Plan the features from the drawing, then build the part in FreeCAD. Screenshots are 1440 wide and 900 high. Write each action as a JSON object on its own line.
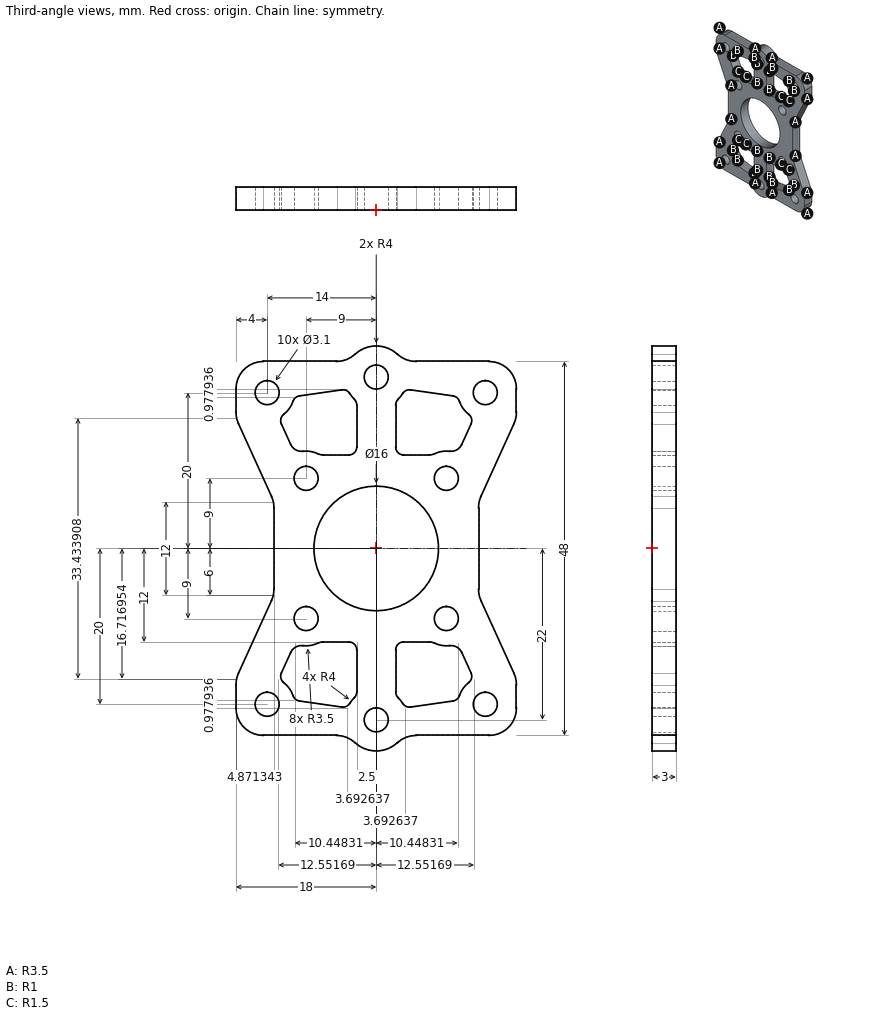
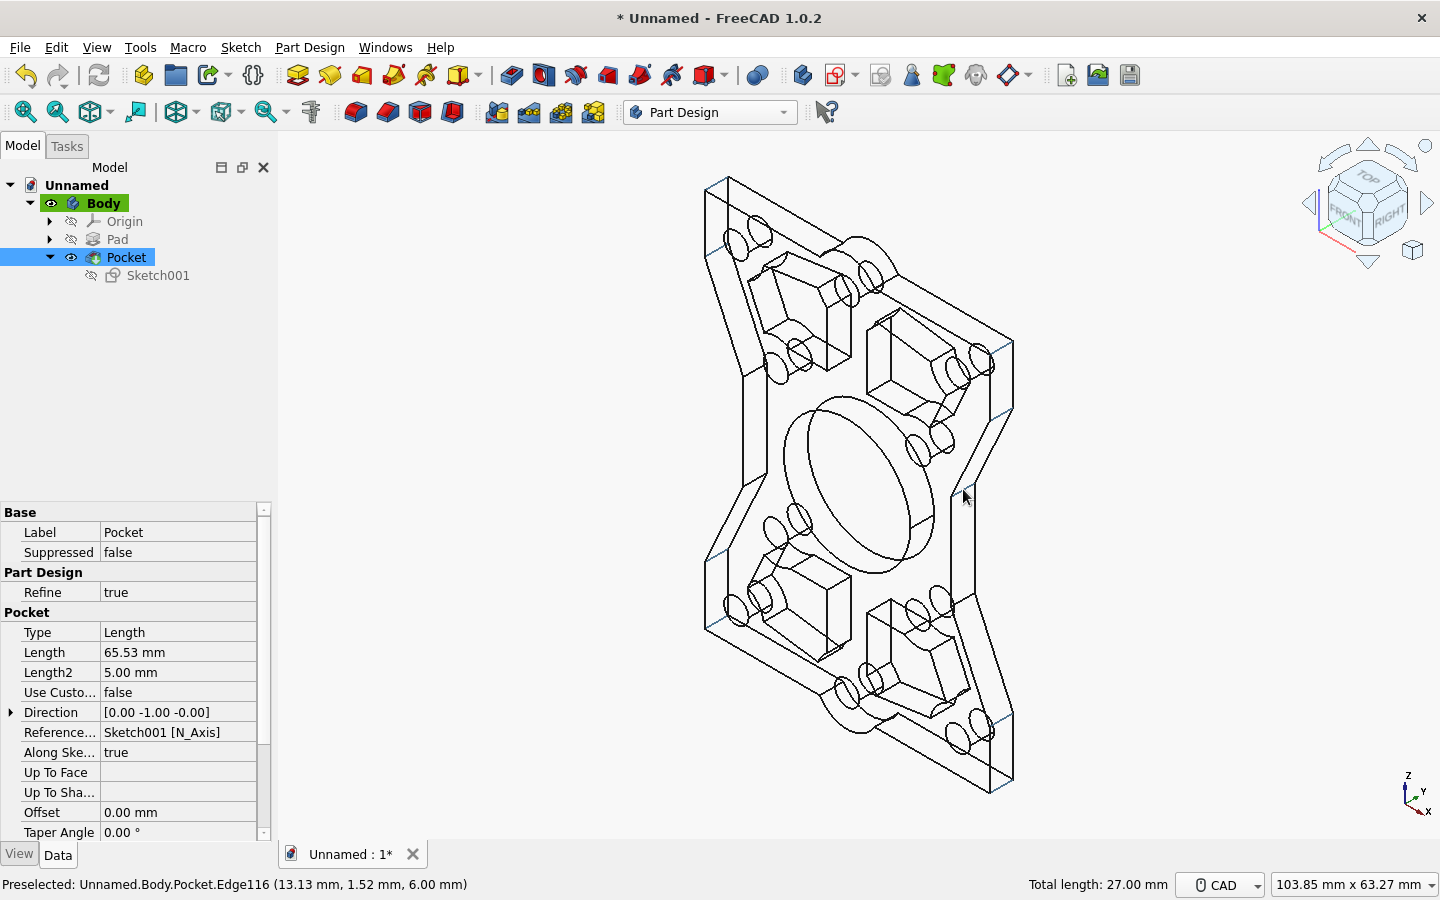
{"action": "left_click", "coordinate": [963, 599], "text": "ctrl"}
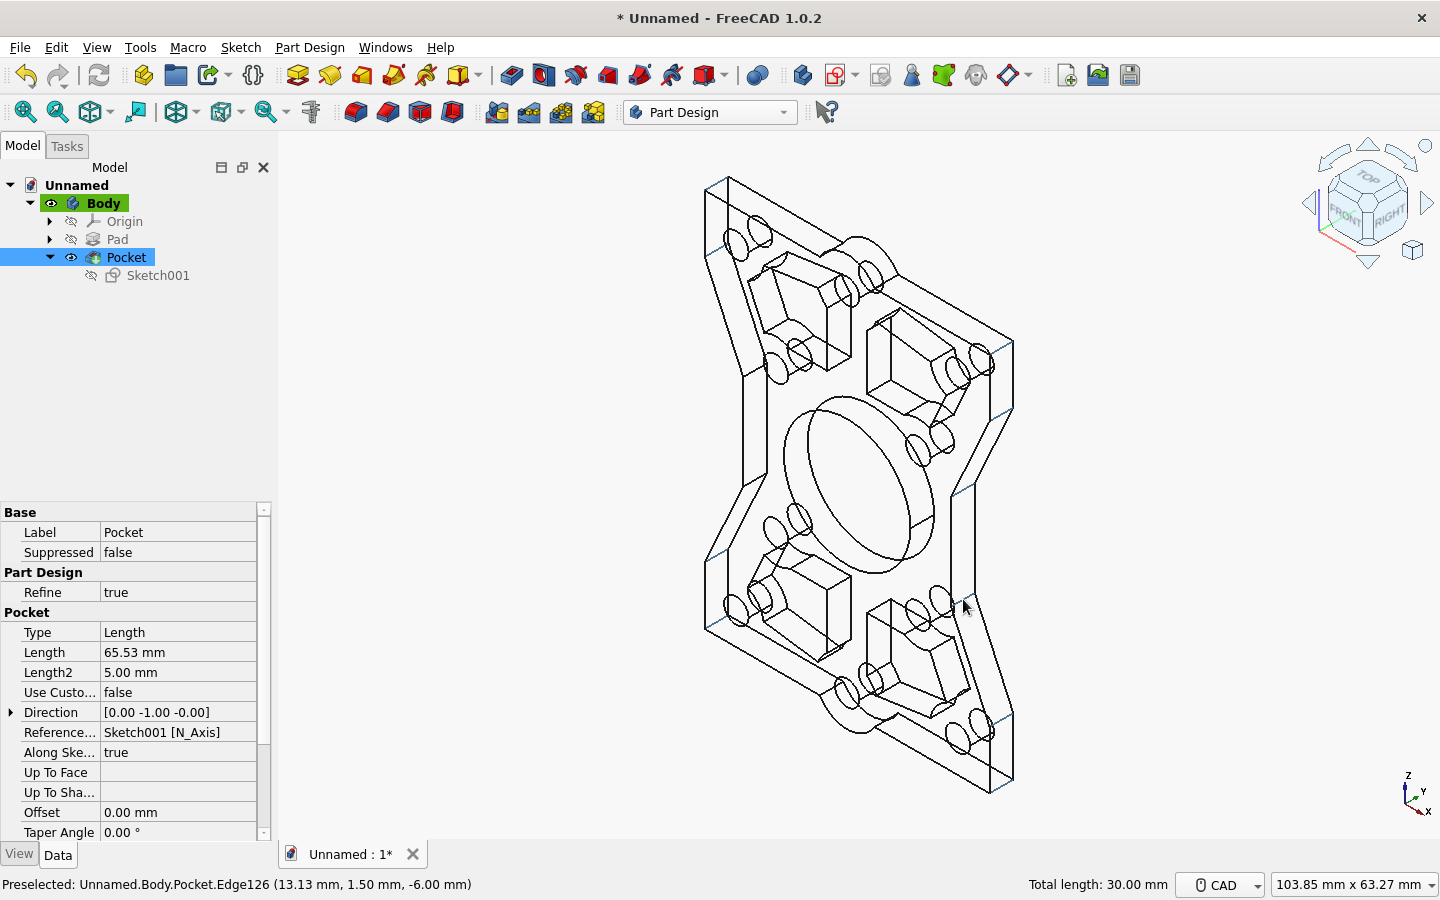
{"action": "left_click", "coordinate": [755, 479], "text": "ctrl"}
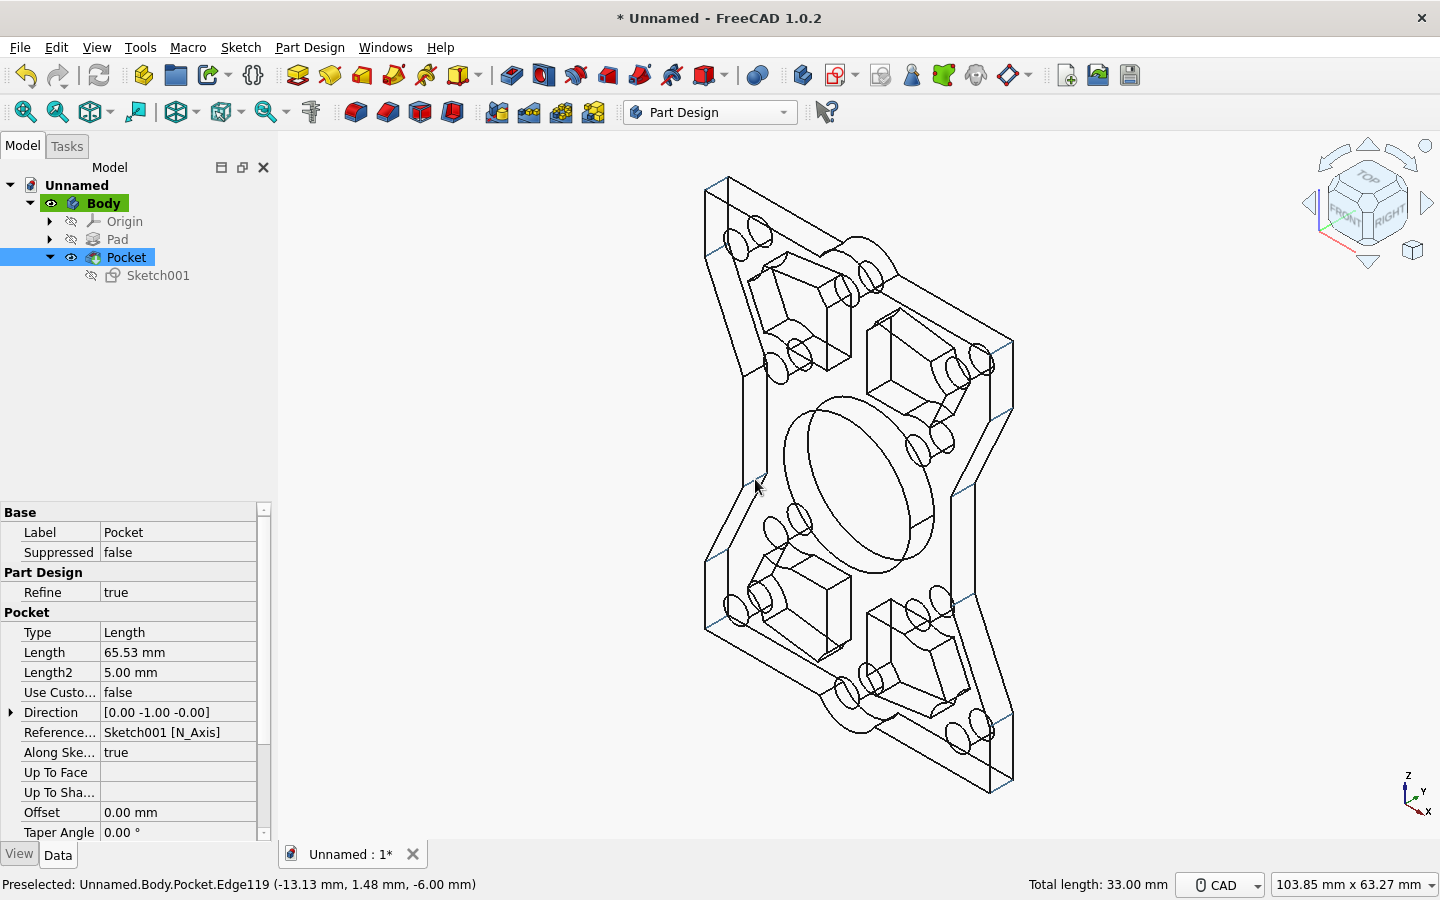
{"action": "left_click", "coordinate": [755, 369], "text": "ctrl"}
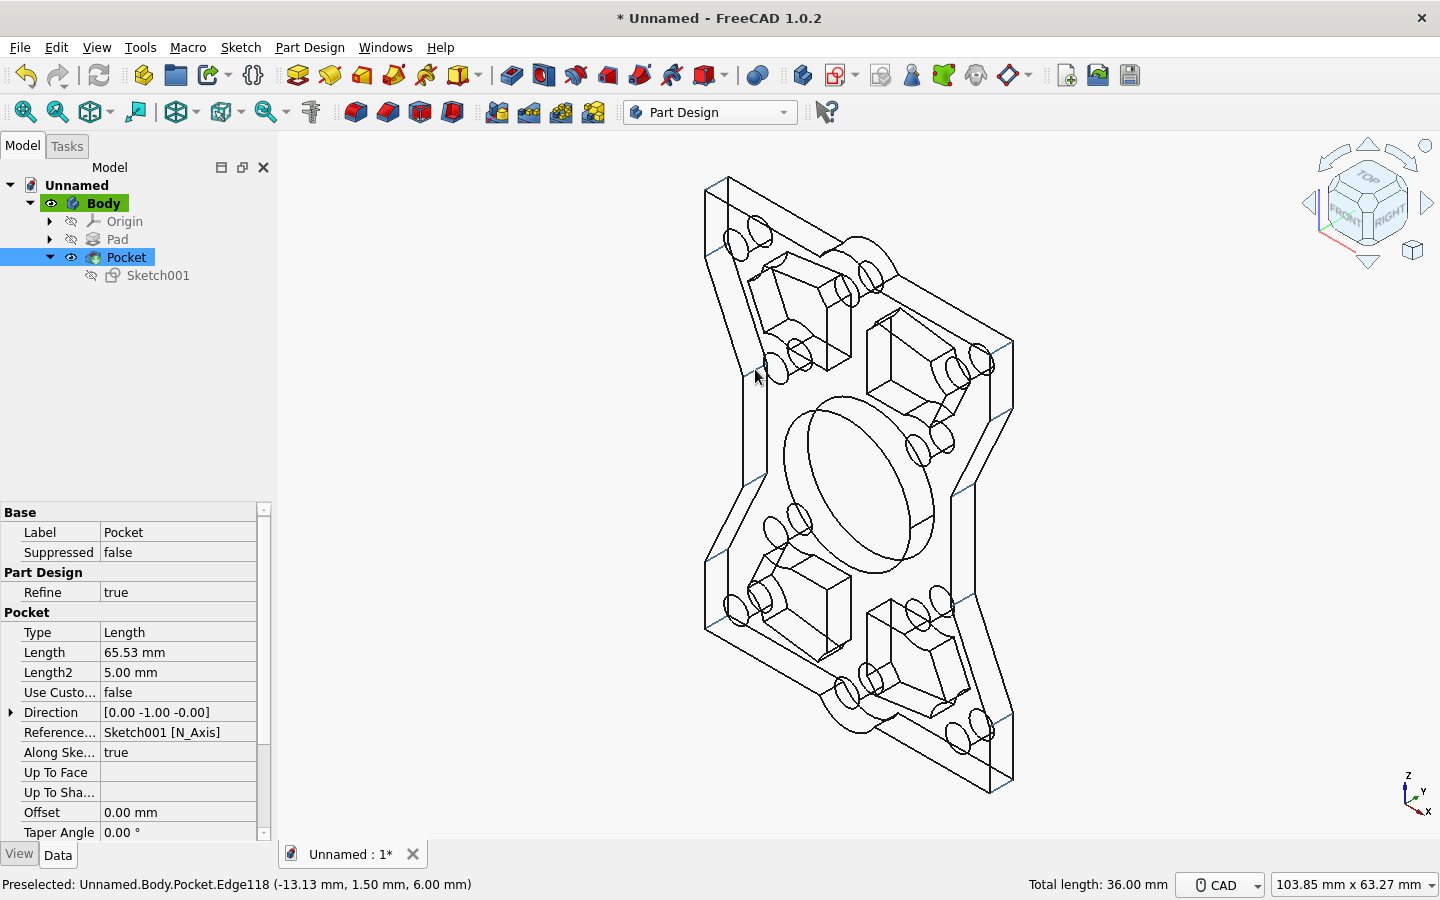
{"action": "left_click", "coordinate": [829, 689], "text": "ctrl"}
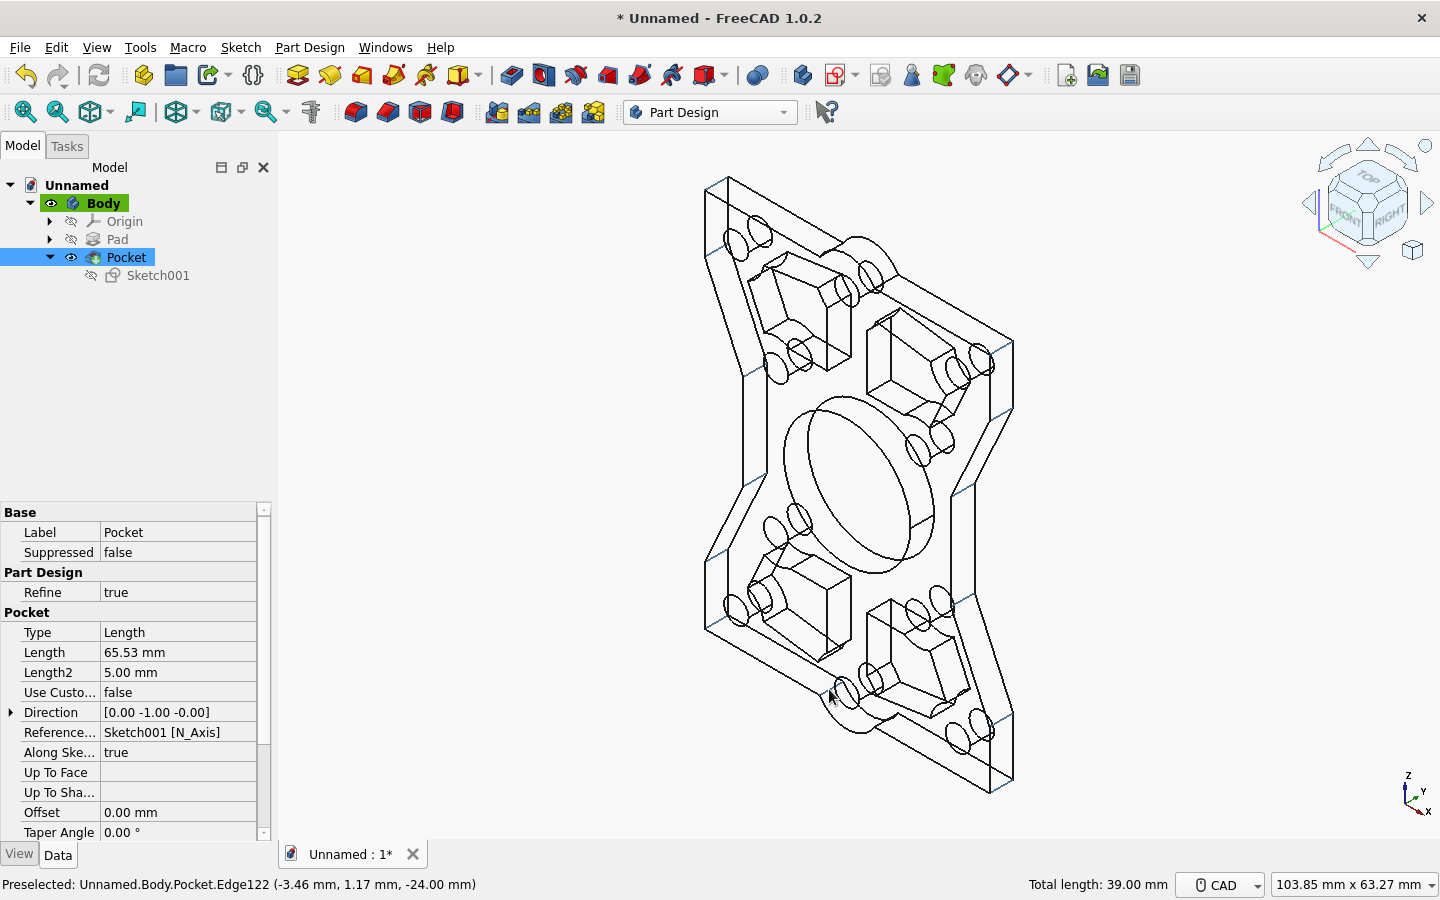
{"action": "left_click", "coordinate": [886, 719], "text": "ctrl"}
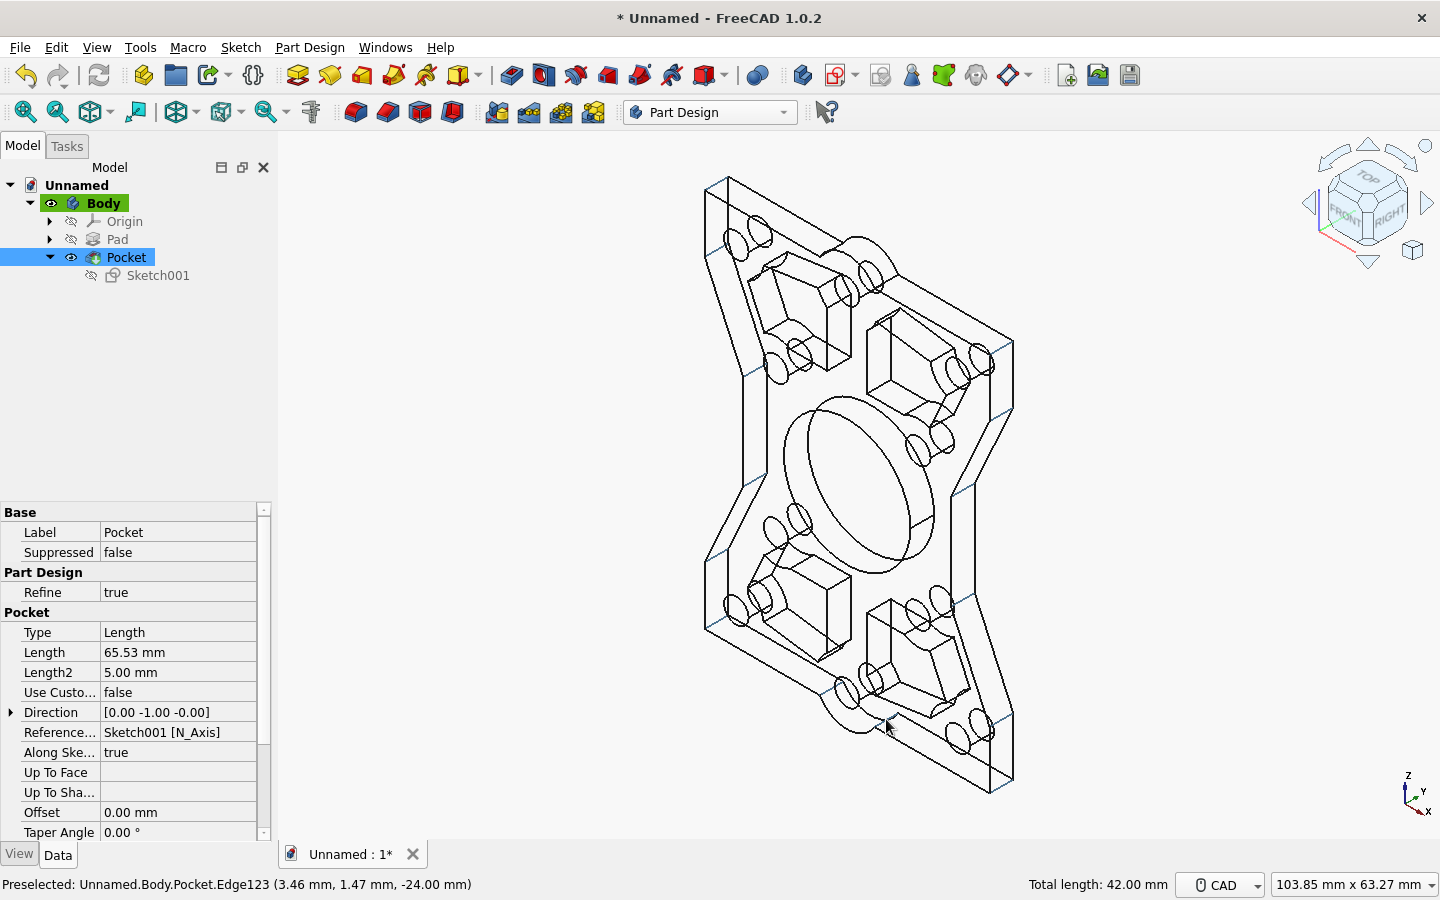
{"action": "left_click", "coordinate": [886, 281], "text": "ctrl"}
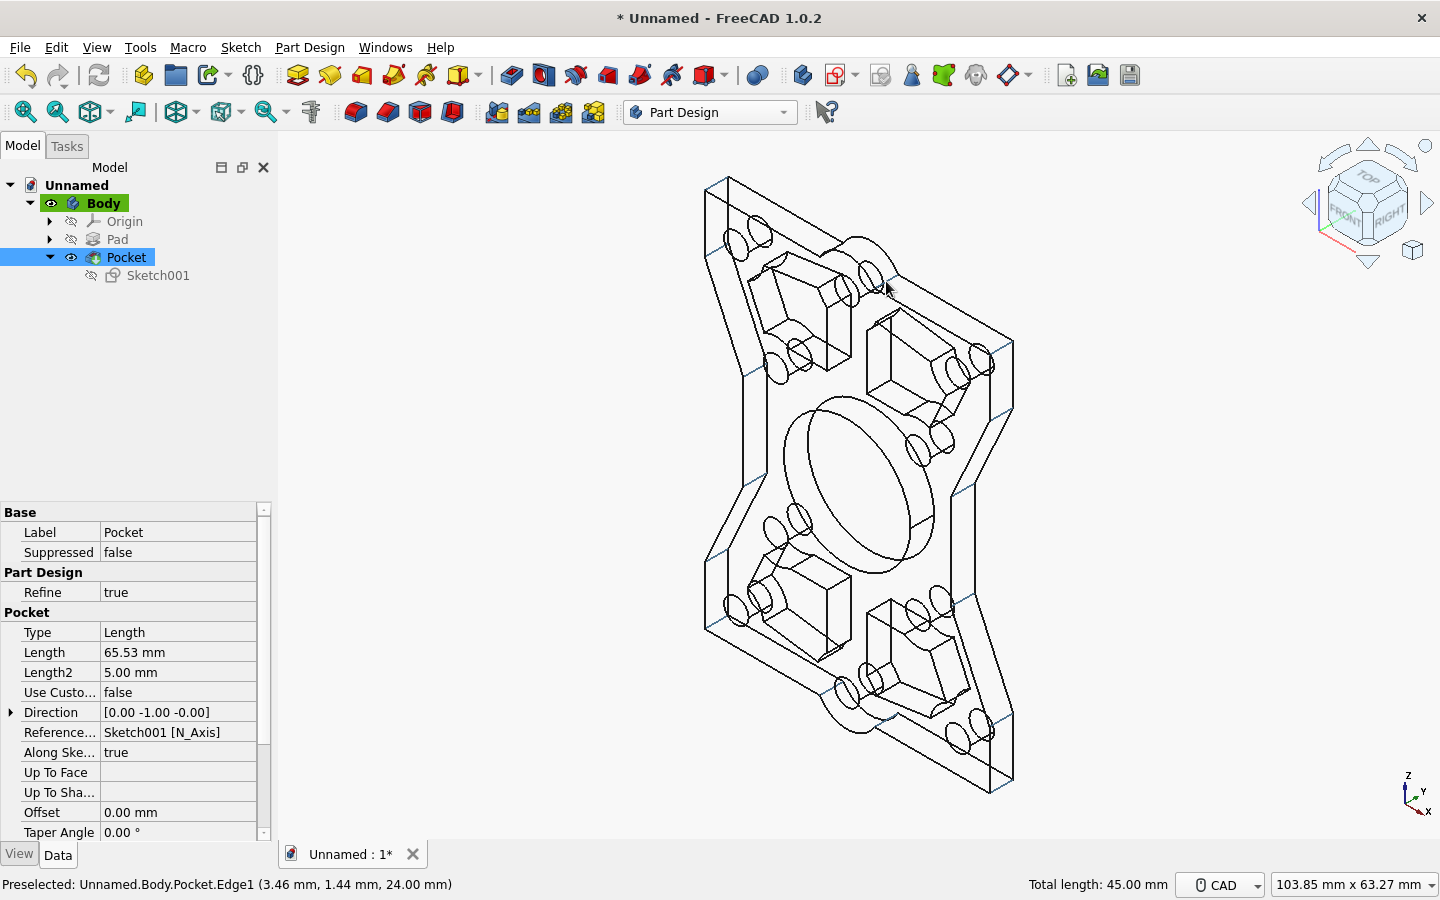
{"action": "key", "text": "2"}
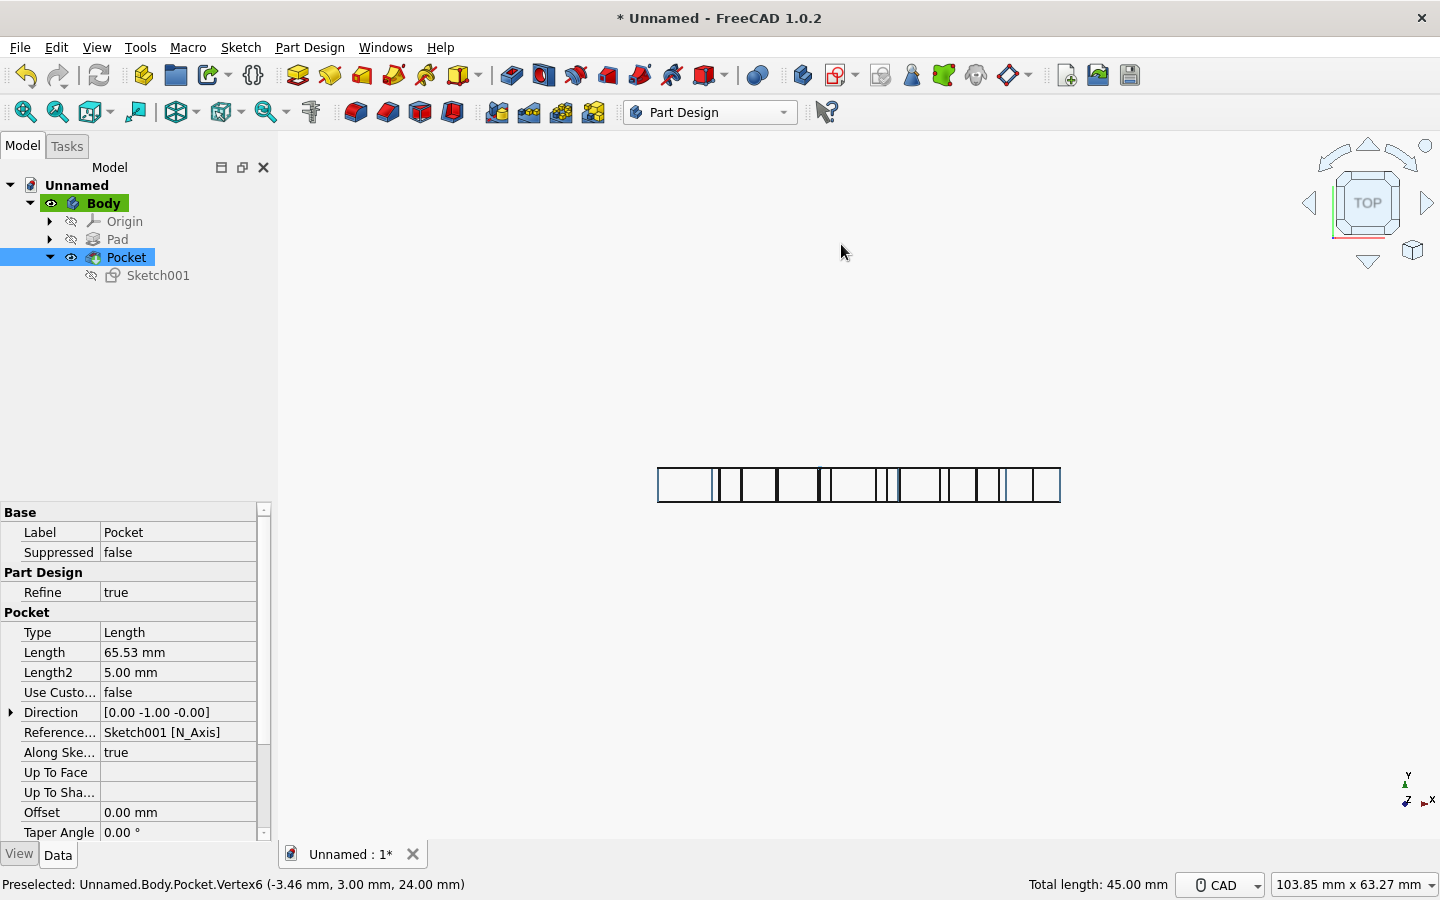
{"action": "left_click", "coordinate": [26, 112]}